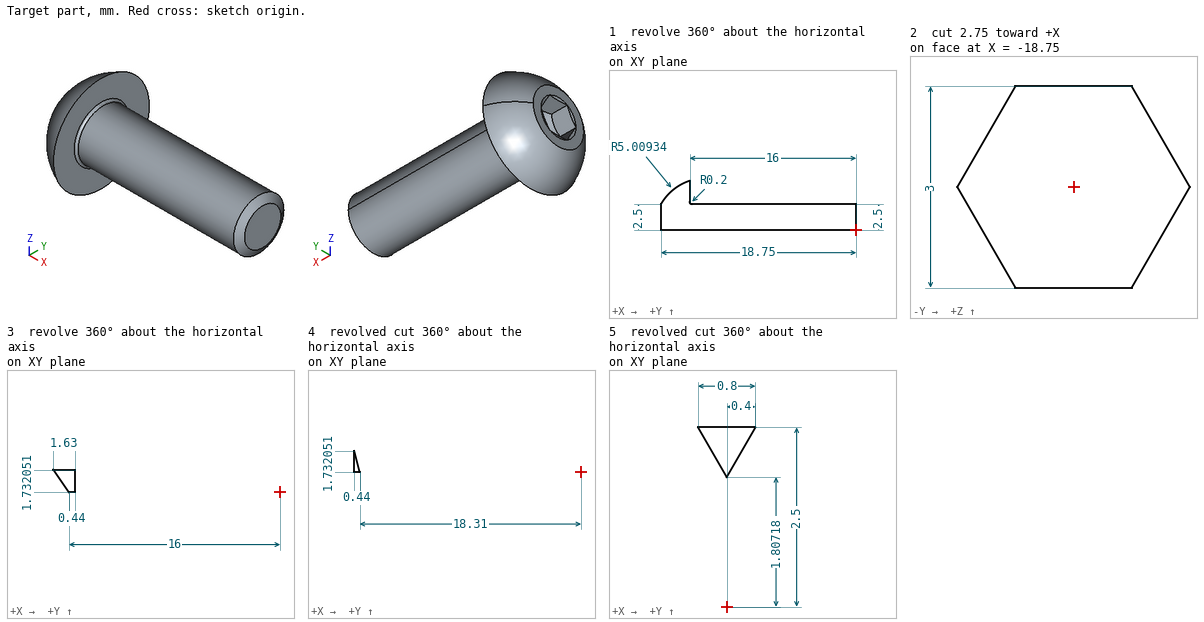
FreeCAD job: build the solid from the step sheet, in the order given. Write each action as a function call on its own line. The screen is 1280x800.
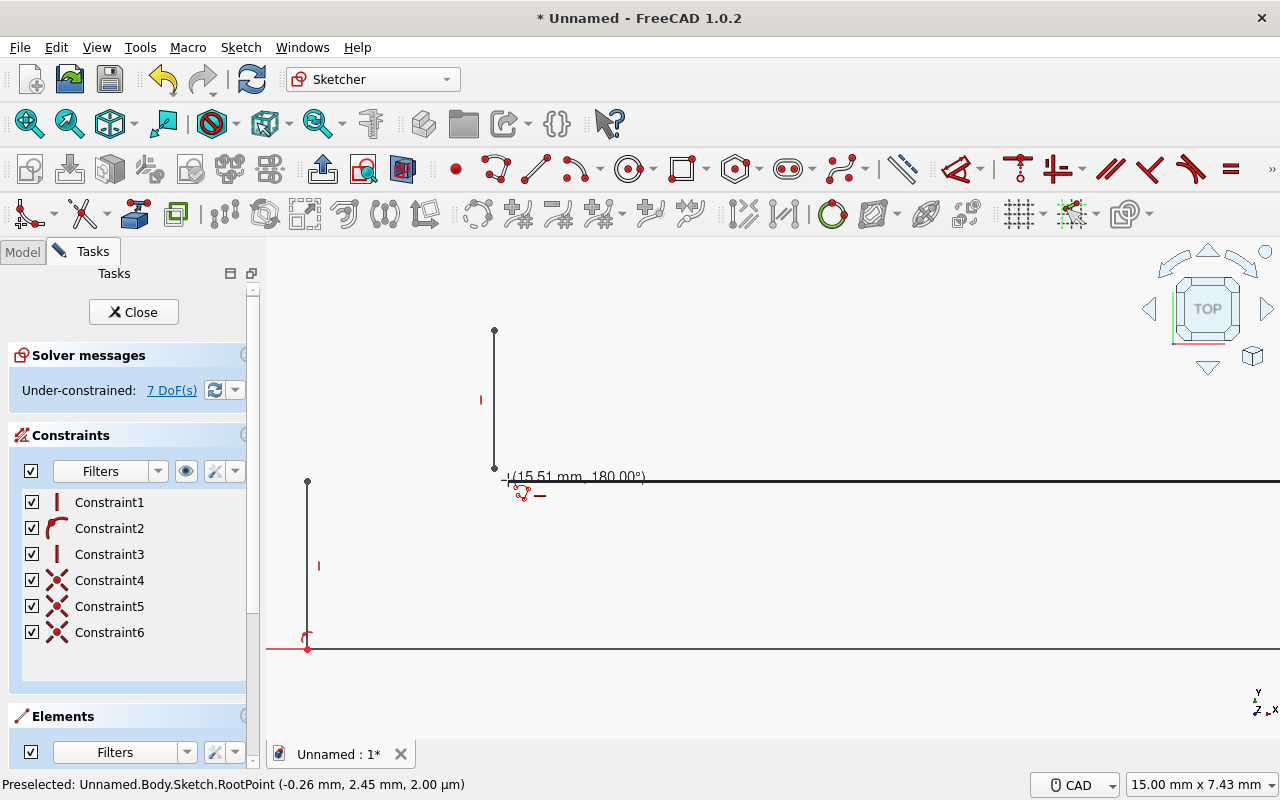
click(508, 479)
right_click(508, 479)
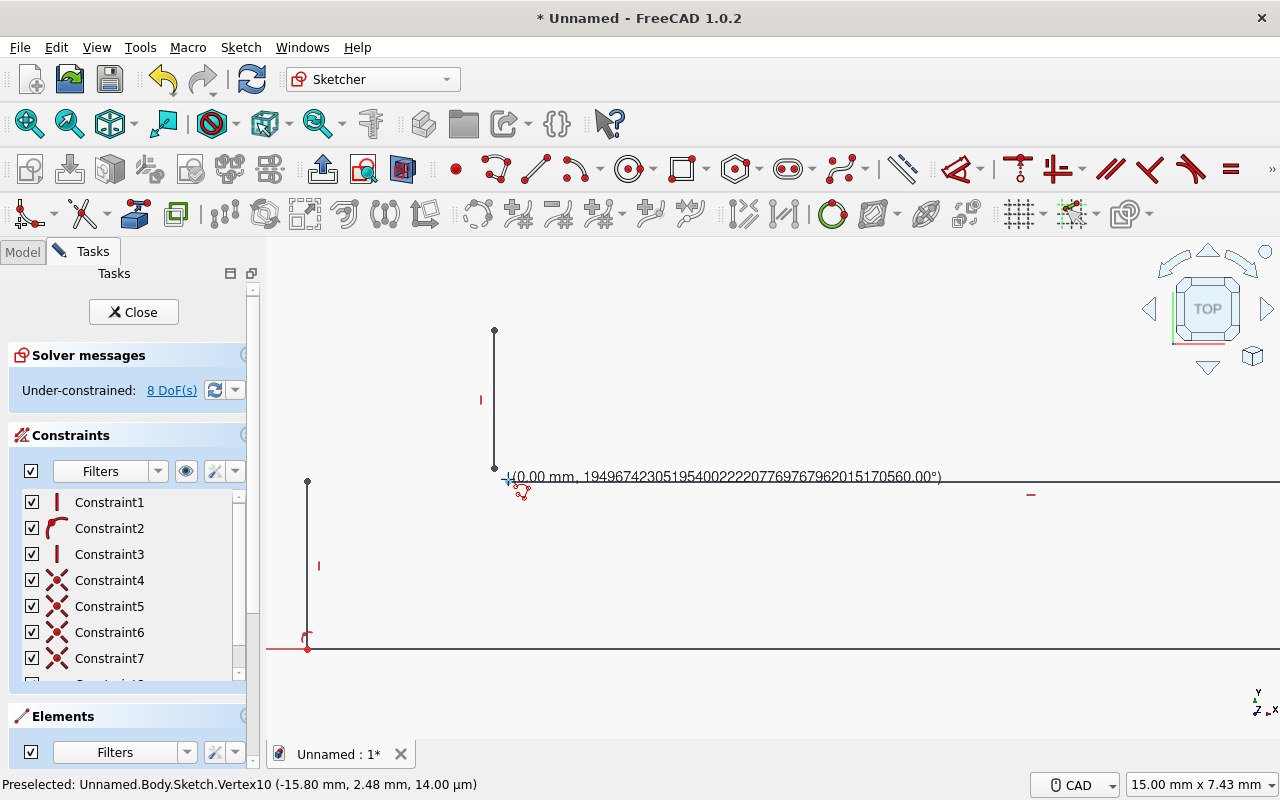
click(602, 170)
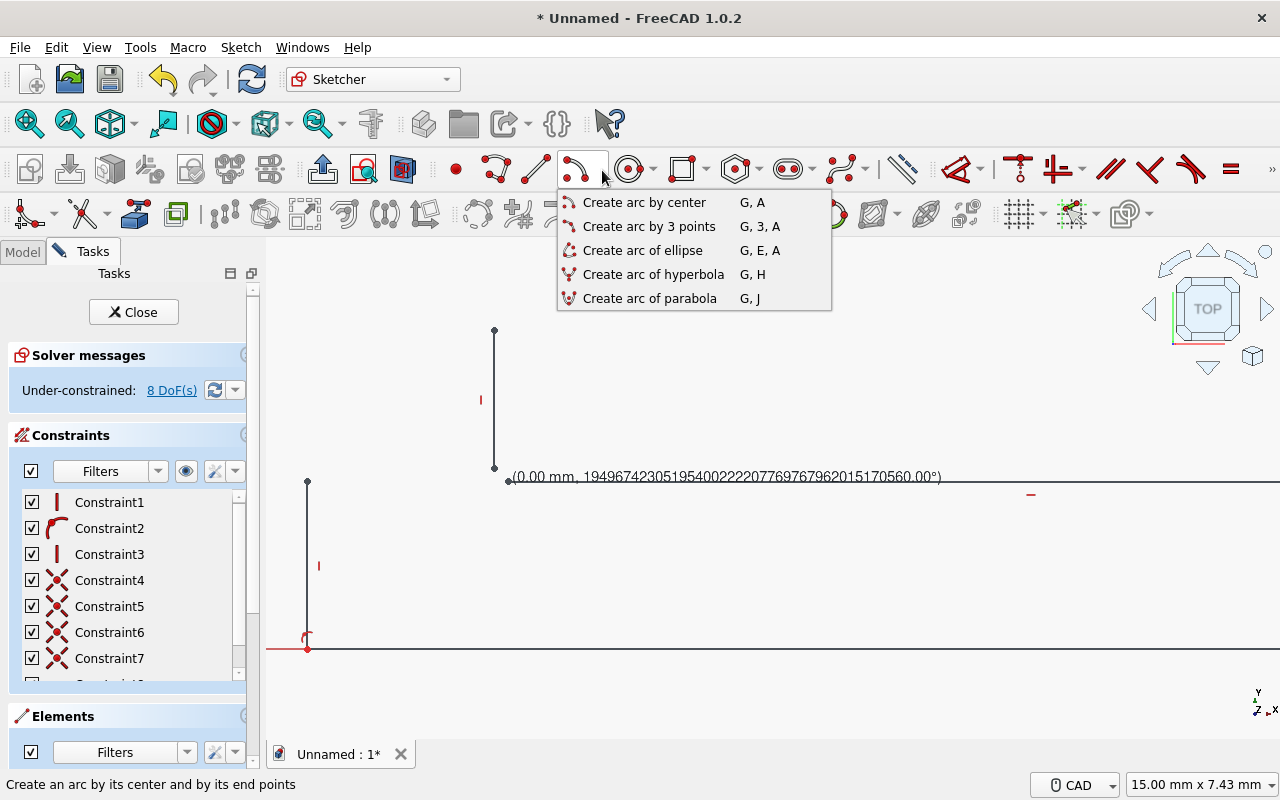
click(694, 226)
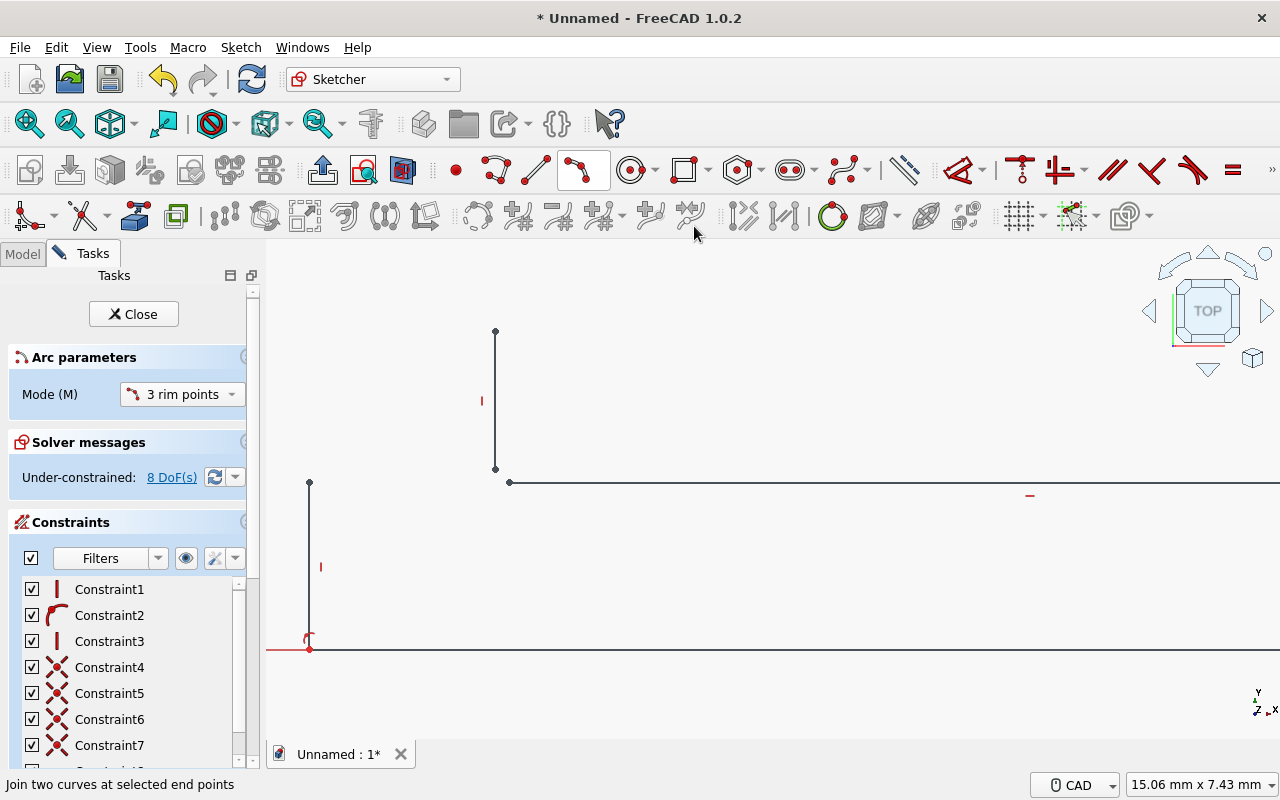
click(495, 332)
click(309, 483)
click(389, 389)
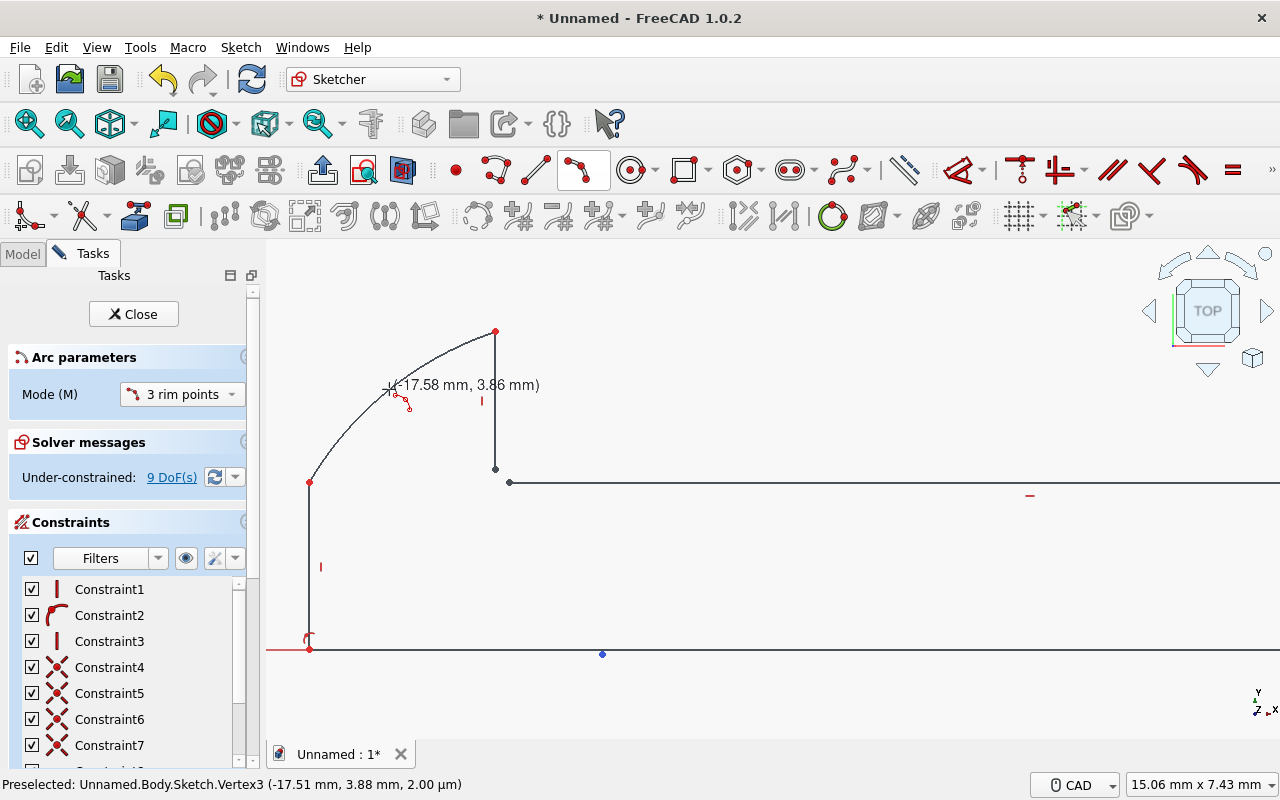
click(509, 483)
click(495, 469)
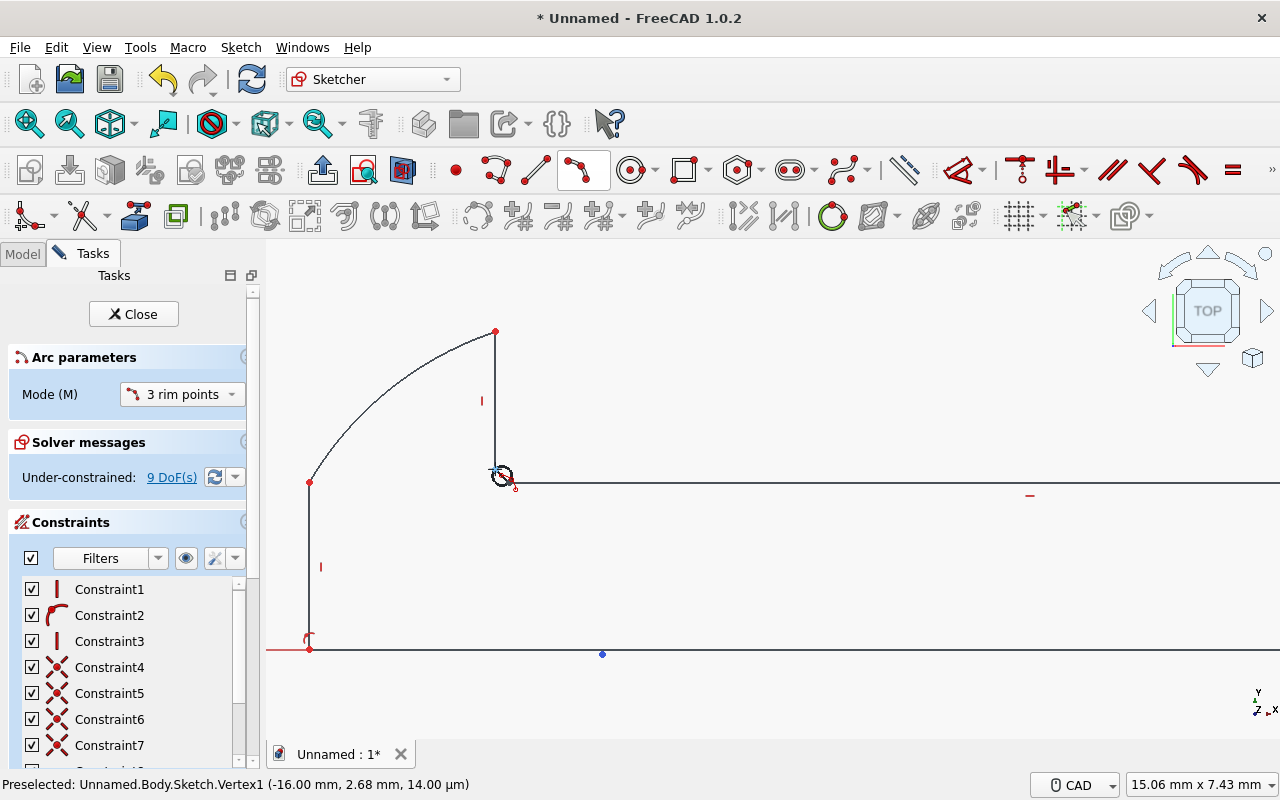
scroll(499, 477, up, 7)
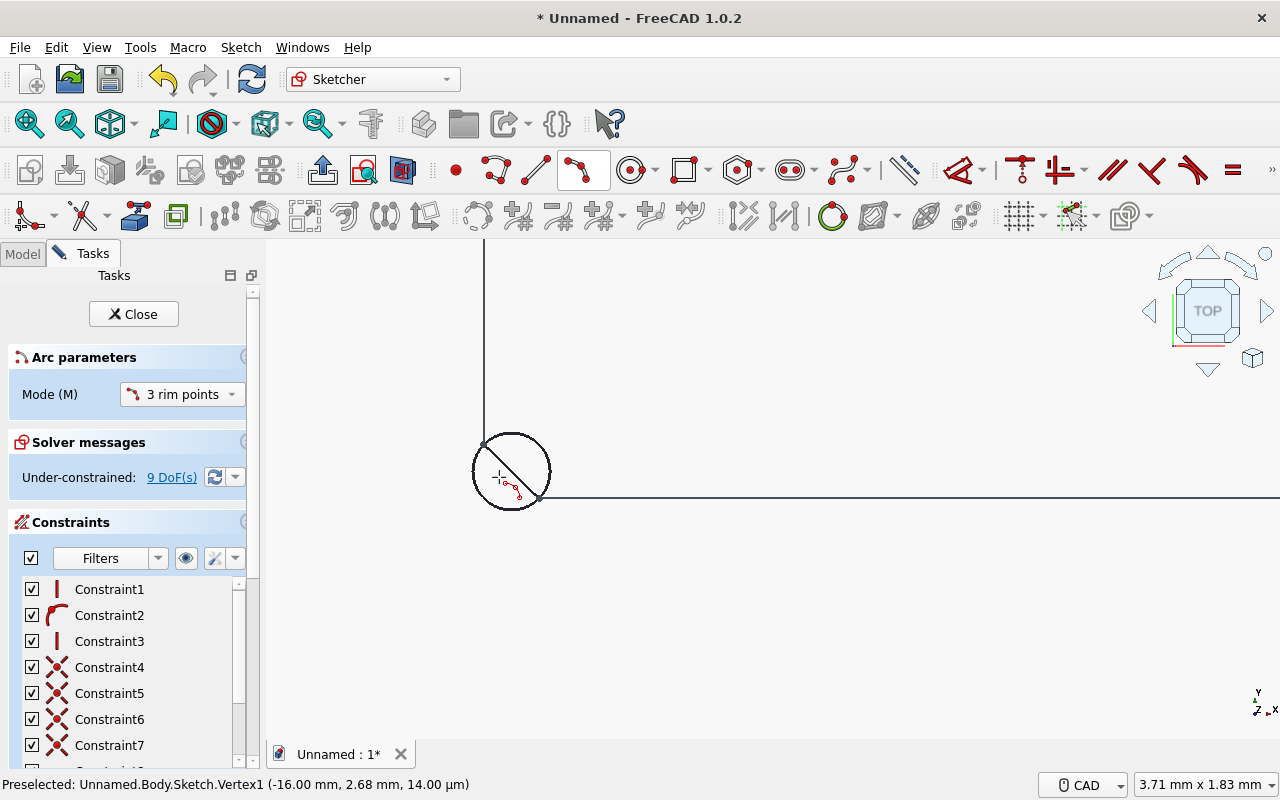
click(499, 477)
key(Escape)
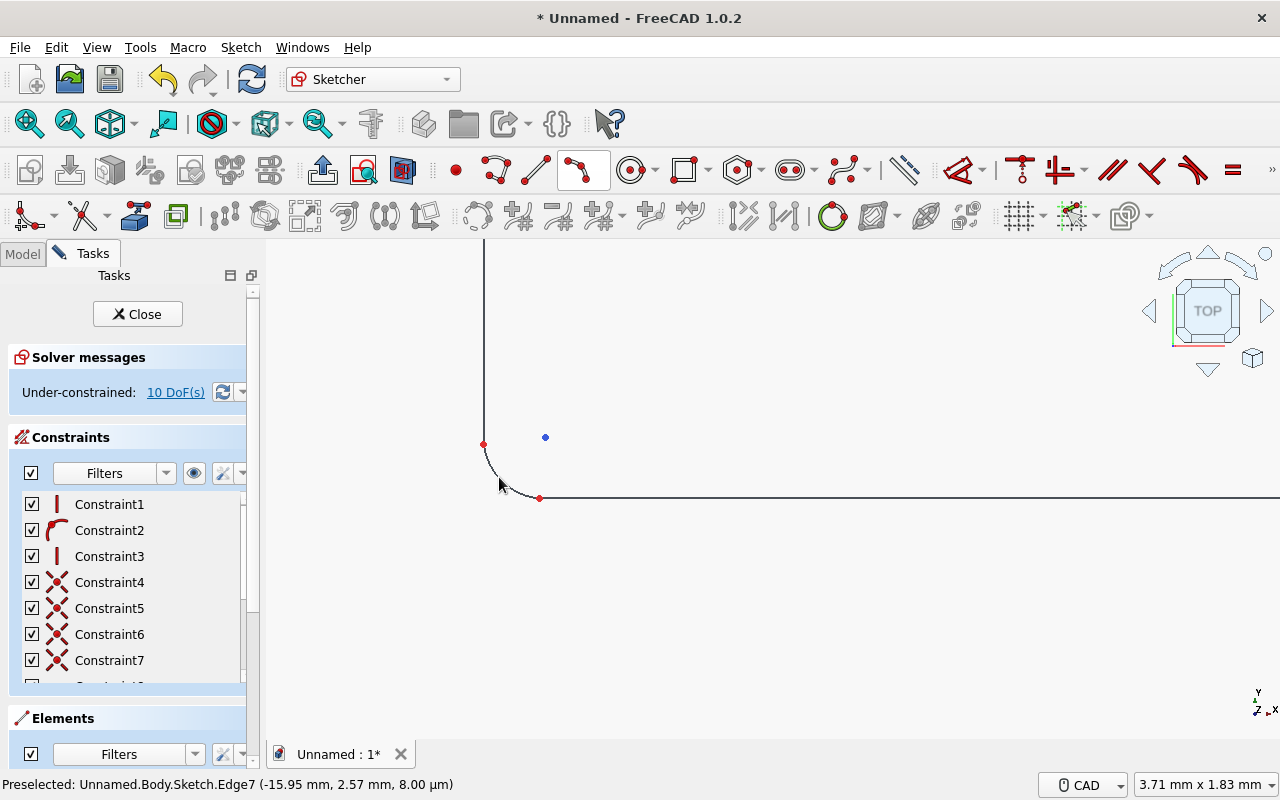
scroll(507, 484, down, 11)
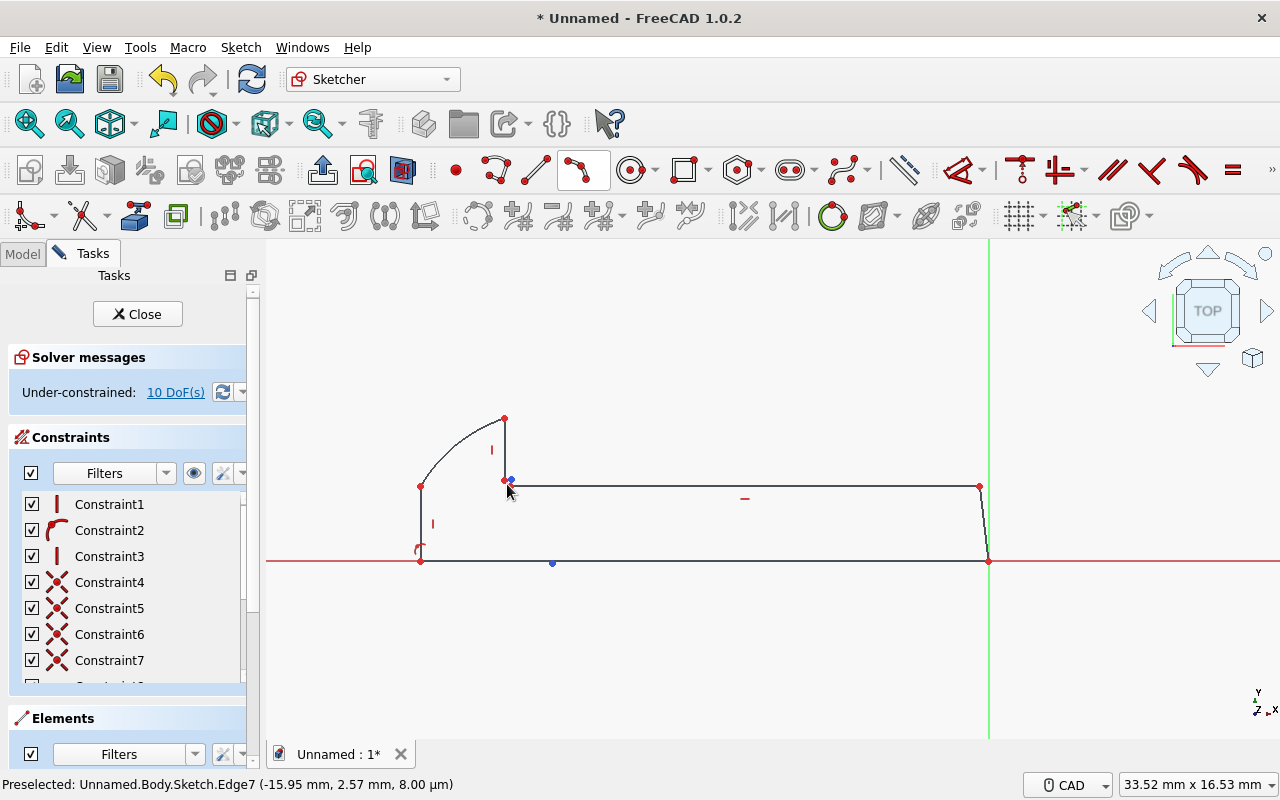
click(505, 462)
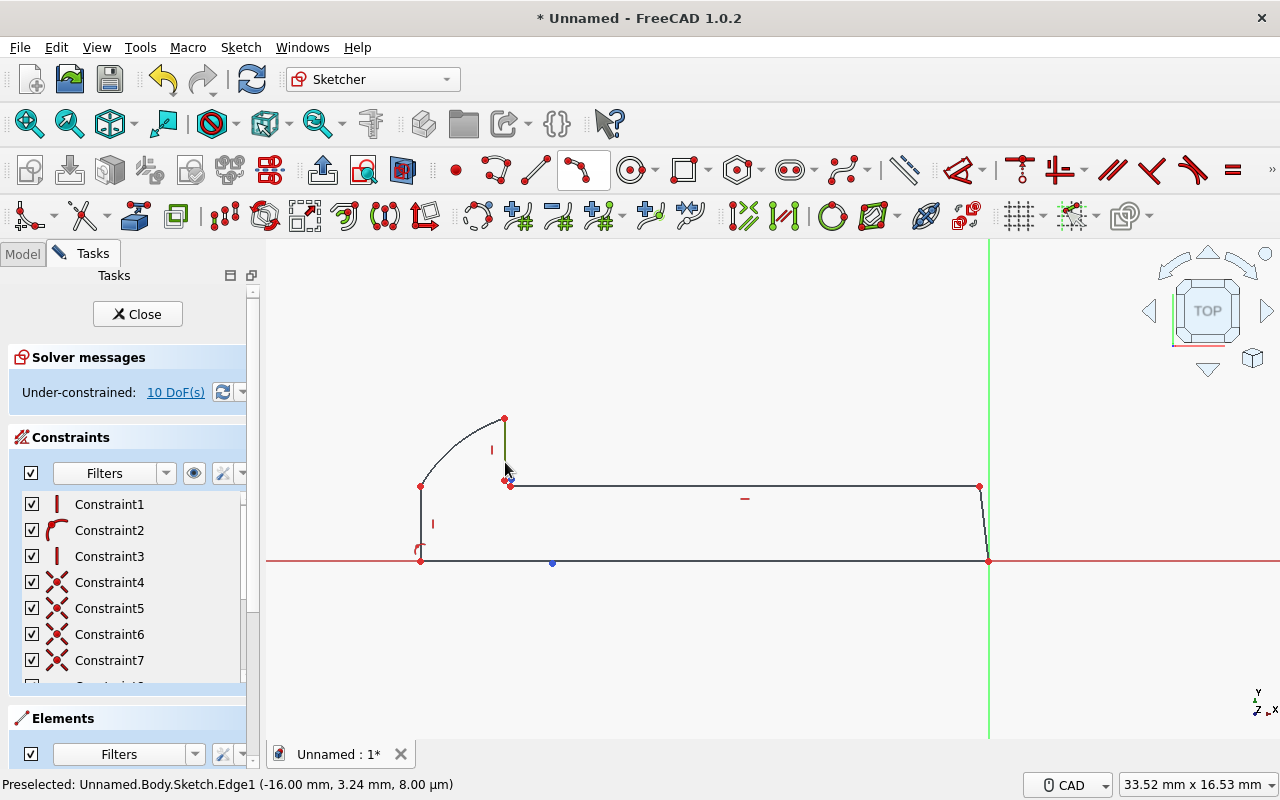
scroll(507, 484, up, 6)